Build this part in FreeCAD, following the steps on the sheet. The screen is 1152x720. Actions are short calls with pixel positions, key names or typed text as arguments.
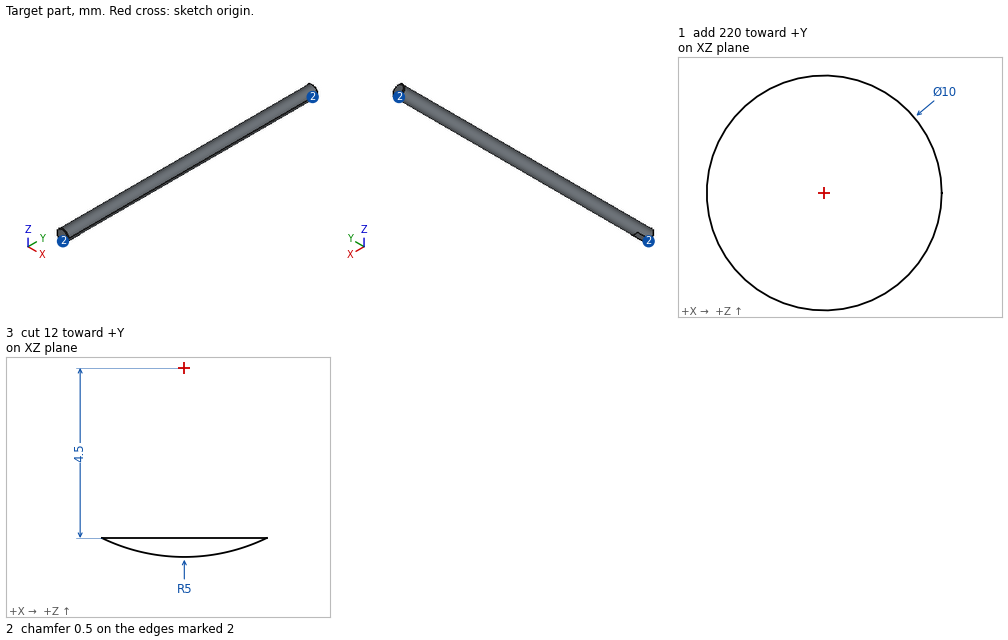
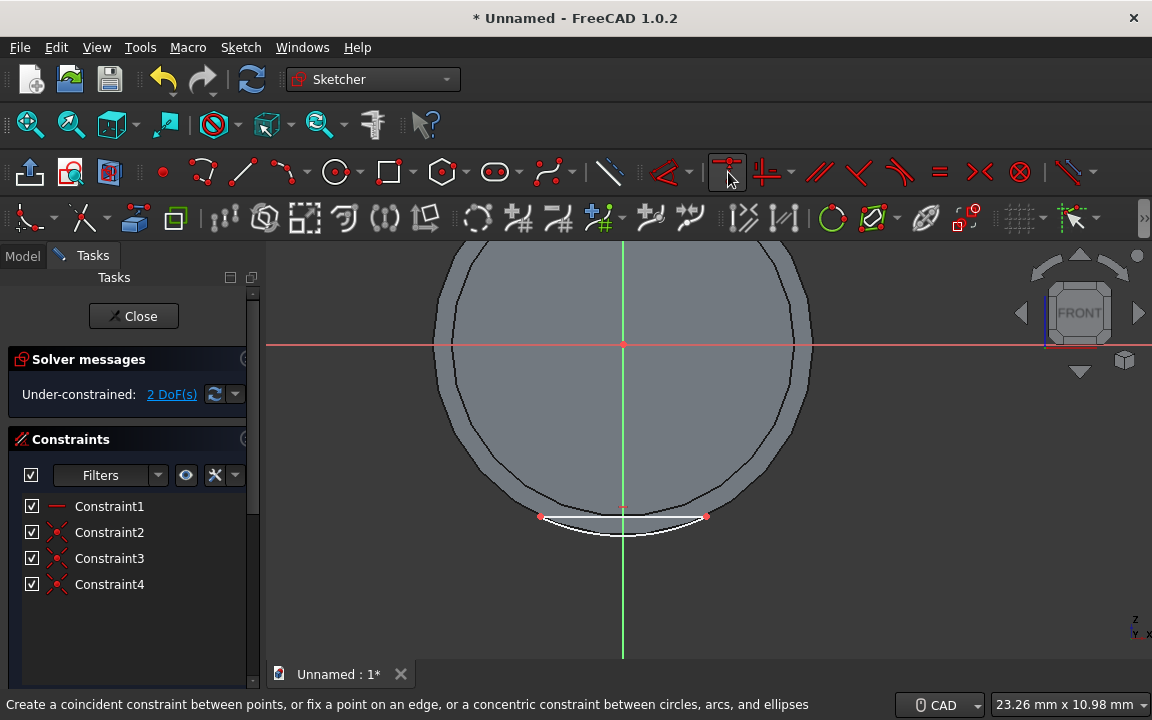
click(664, 172)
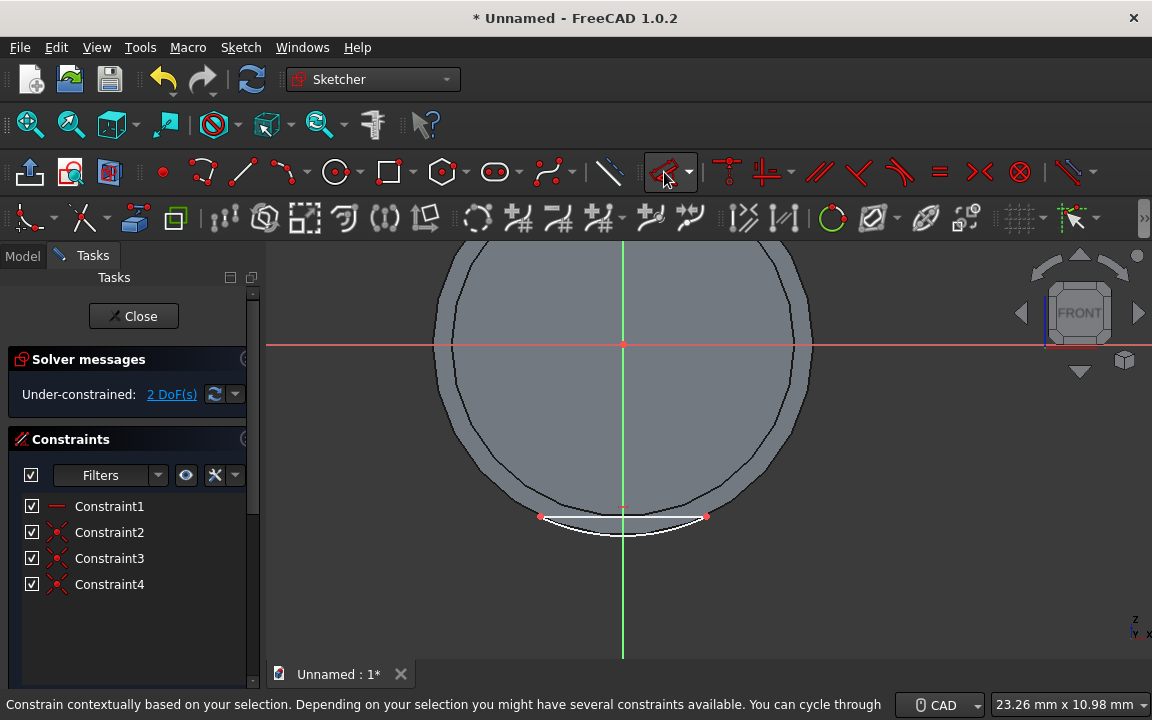
click(589, 533)
click(583, 564)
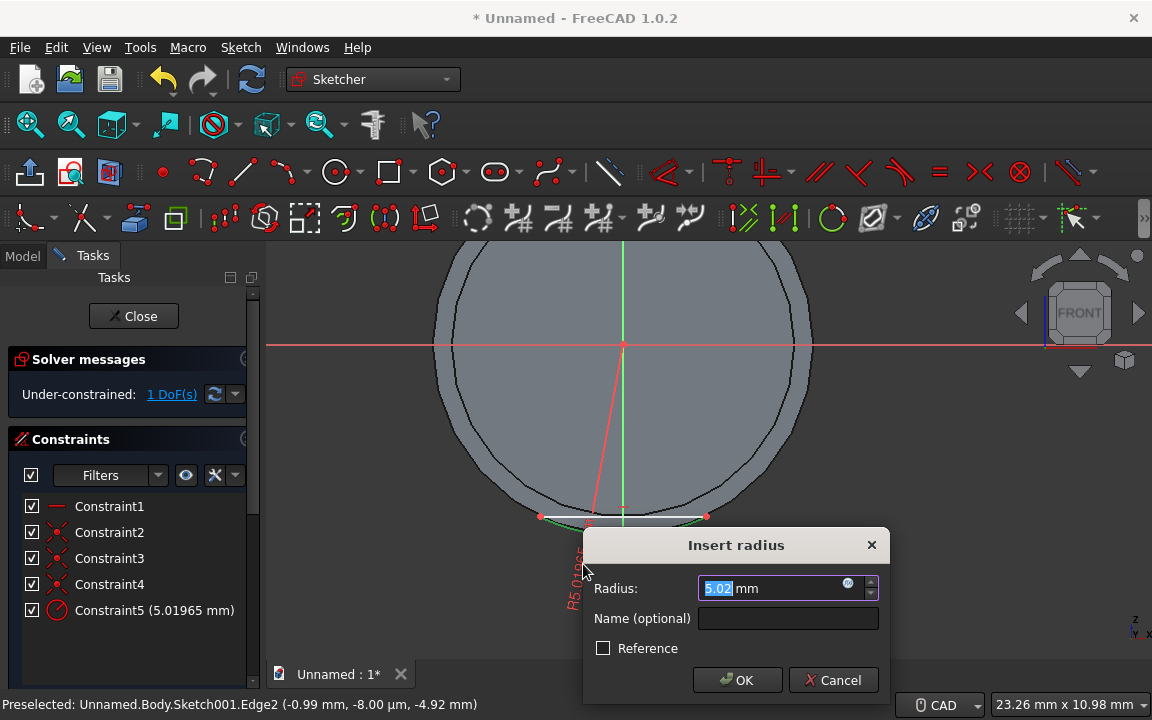
text(5)
key(Return)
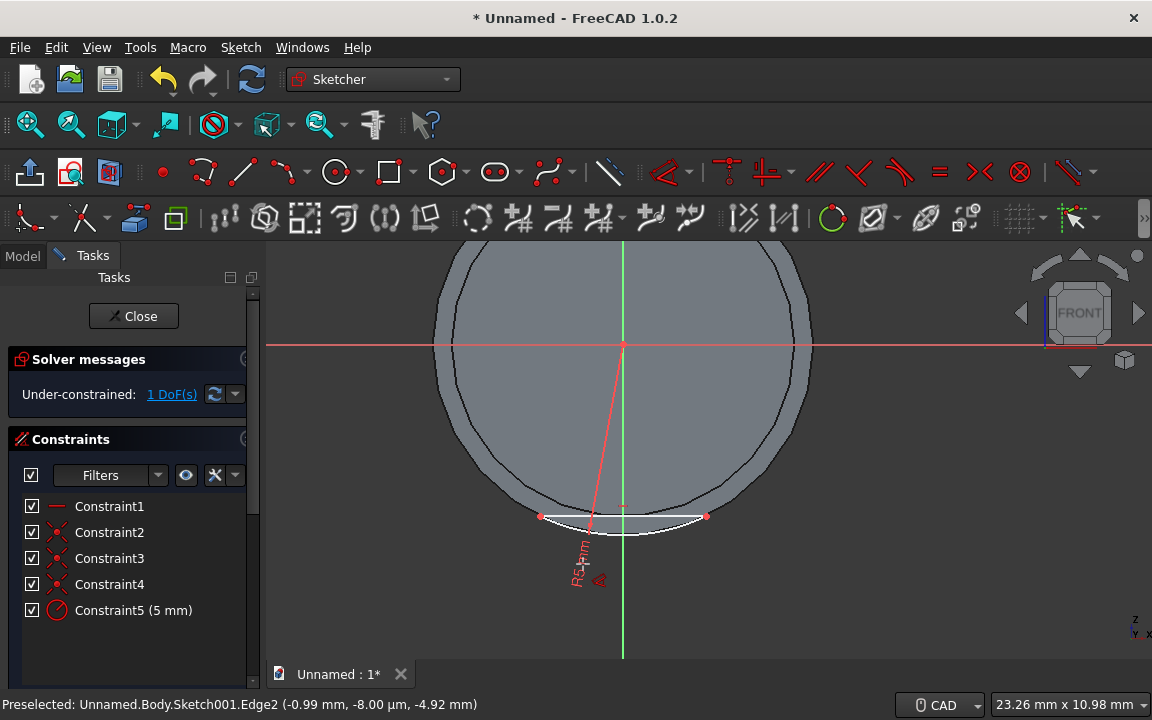
click(540, 516)
click(506, 430)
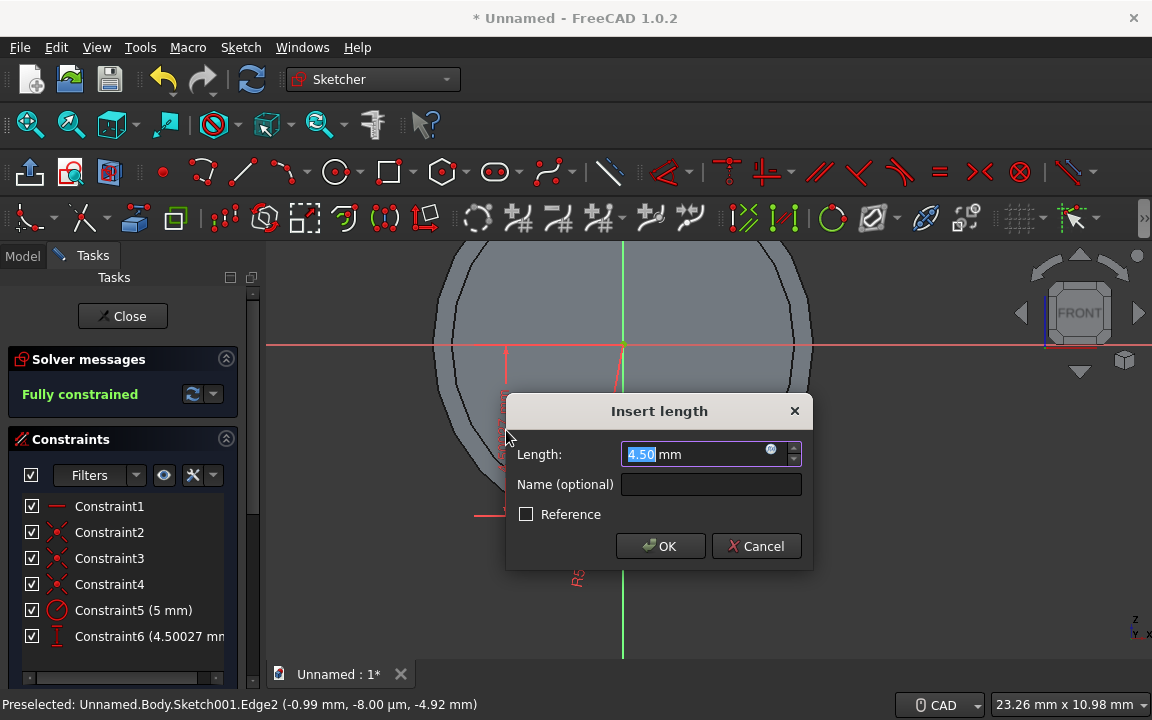
text(4.5)
key(Return)
key(Escape)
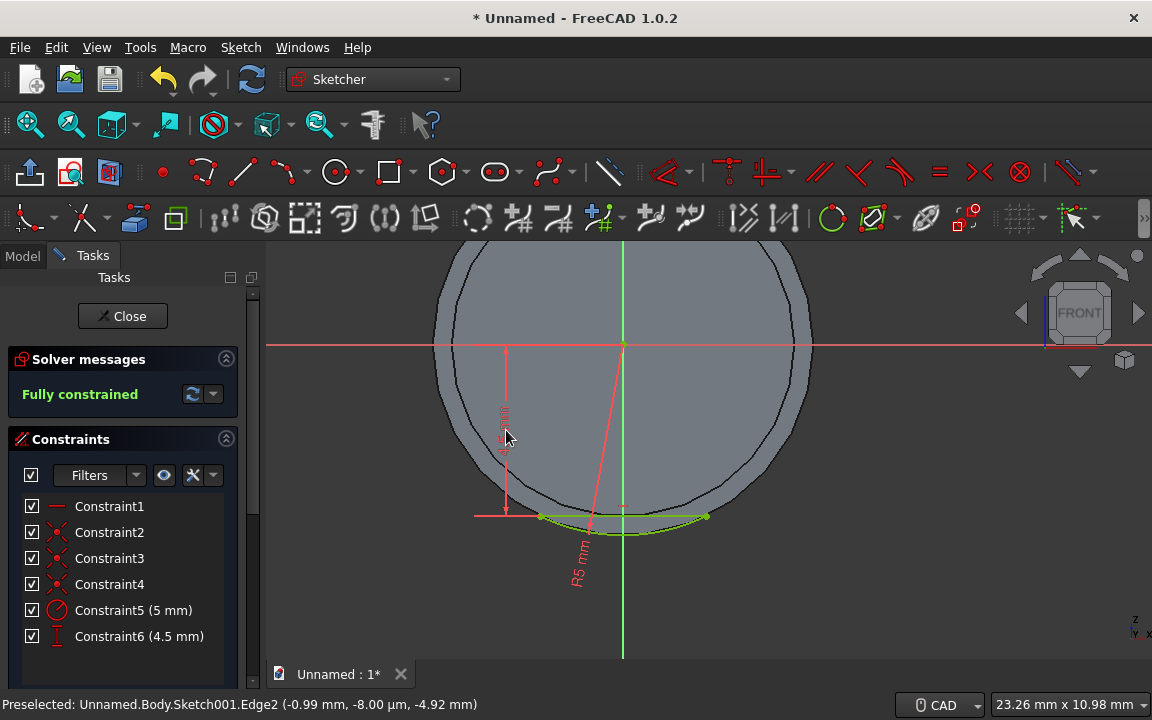
click(123, 316)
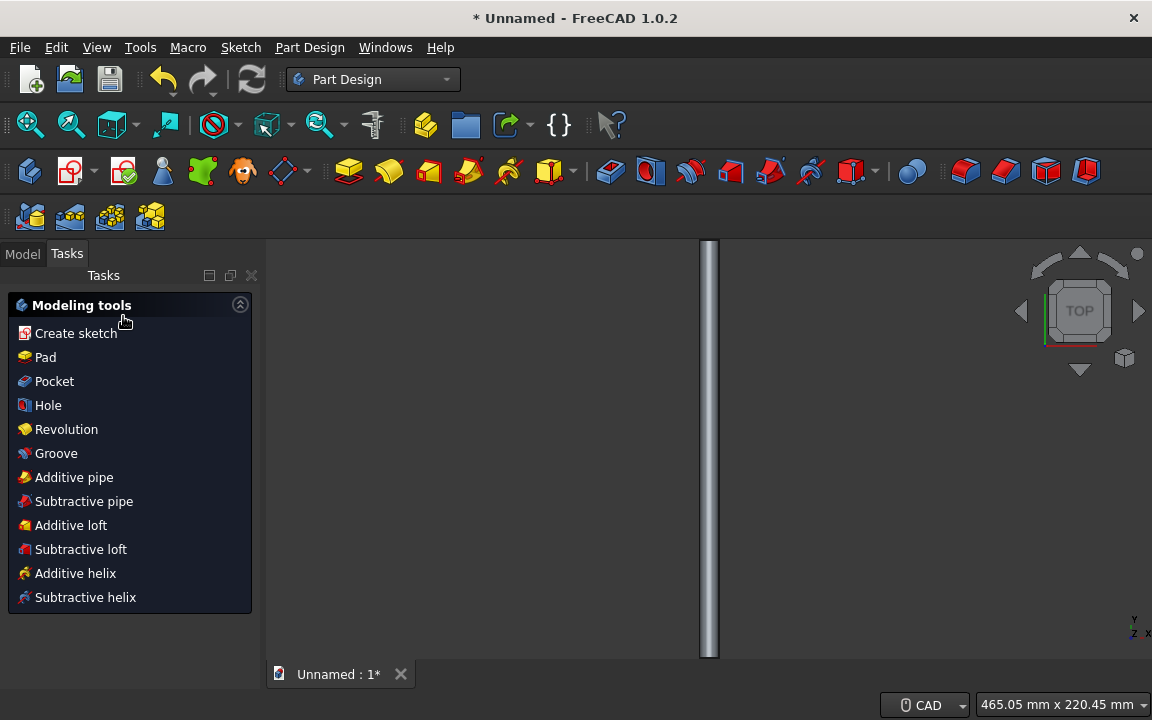
click(612, 172)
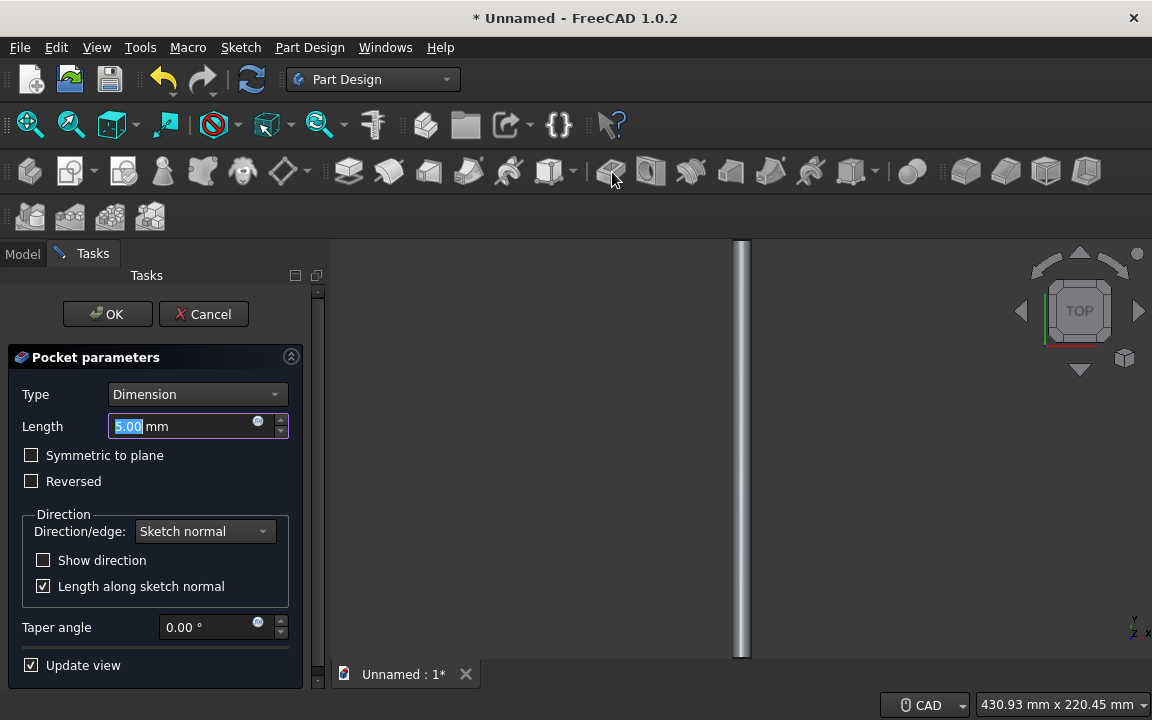
text(12)
key(Tab)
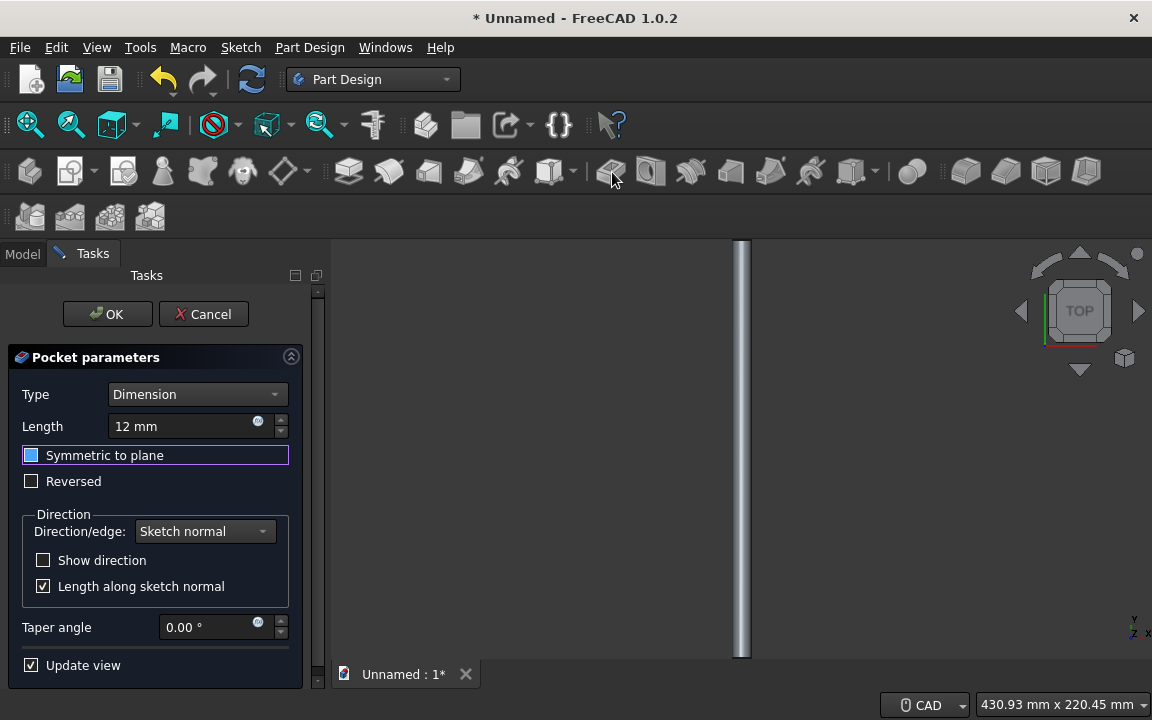
click(108, 314)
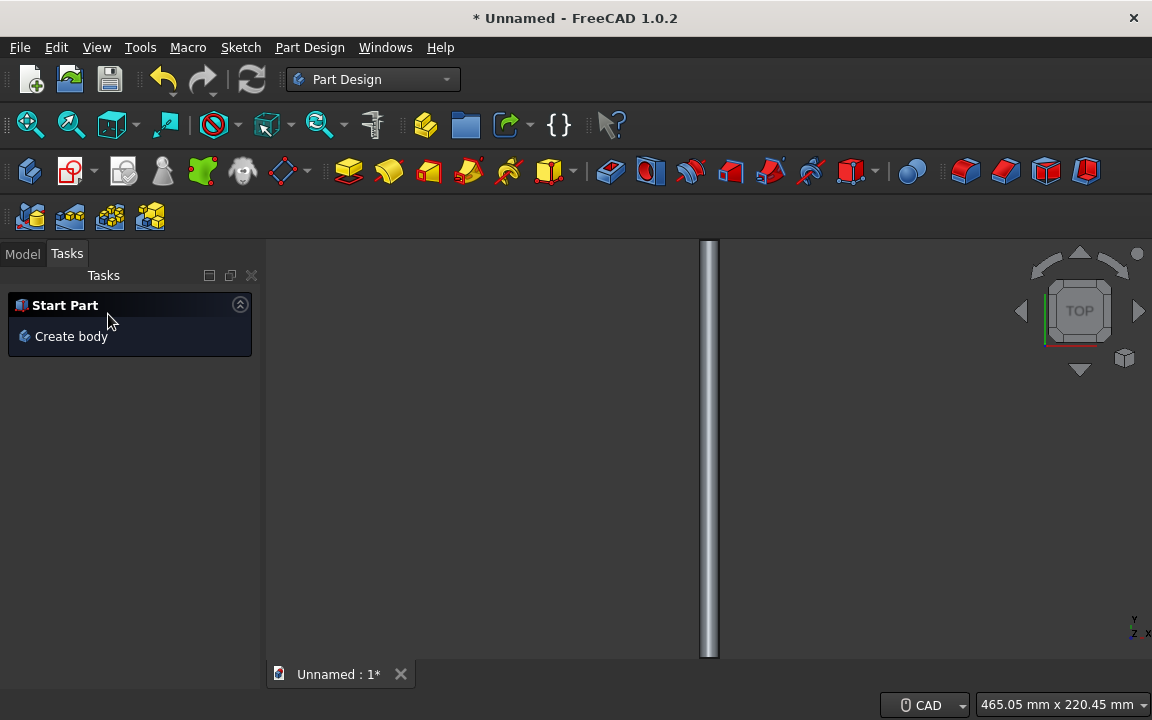
key(0)